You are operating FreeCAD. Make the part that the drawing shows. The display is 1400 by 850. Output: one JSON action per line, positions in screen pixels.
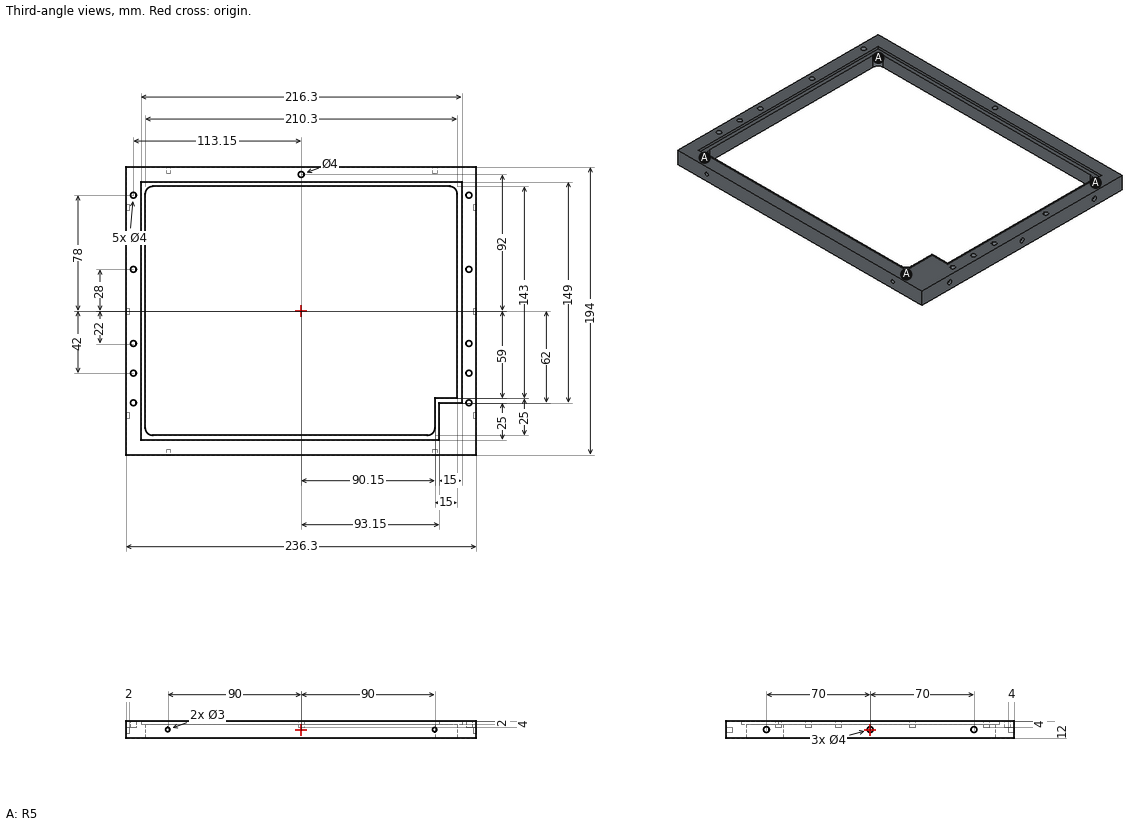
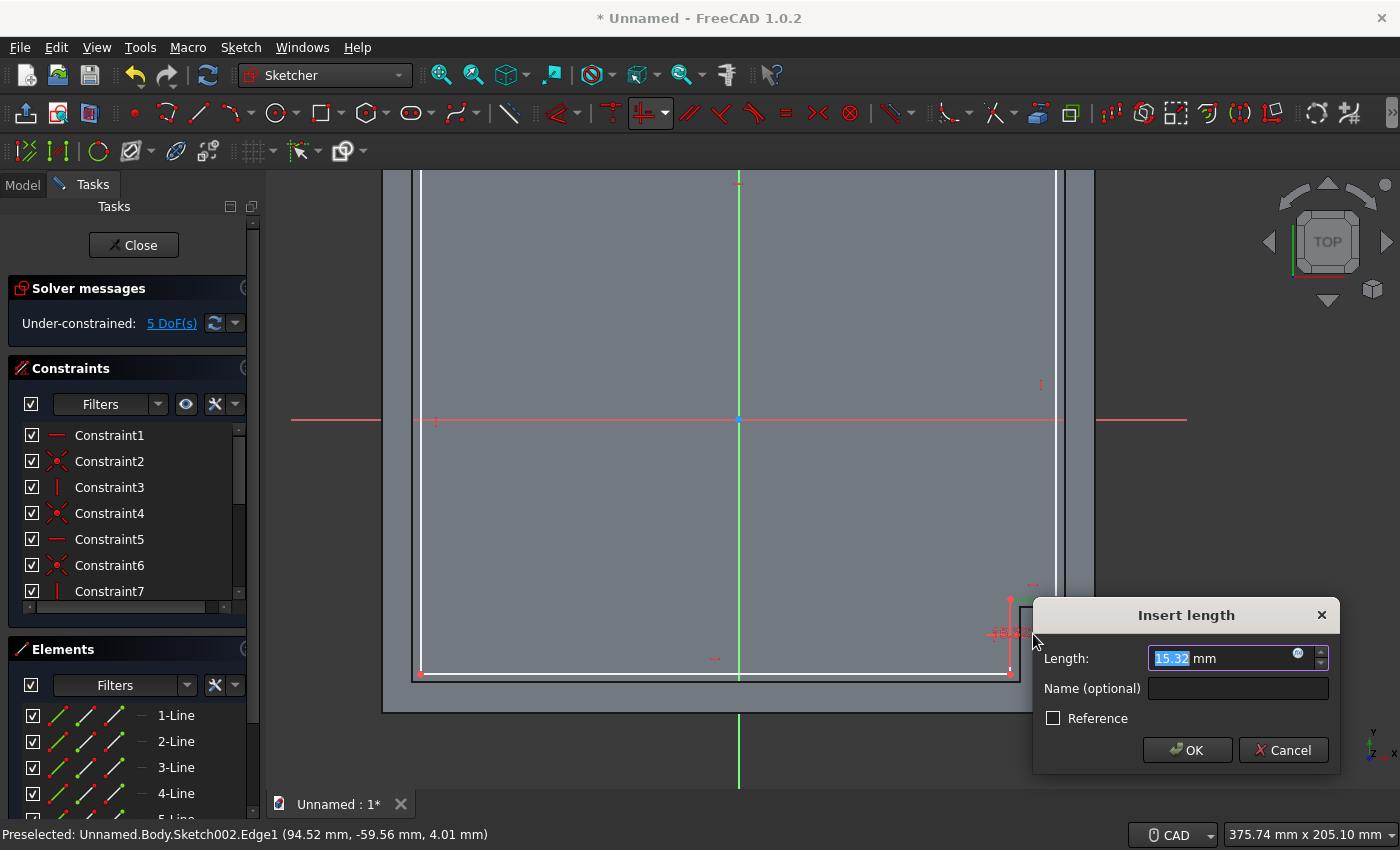
{"action": "type", "text": "15"}
{"action": "key", "text": "Return"}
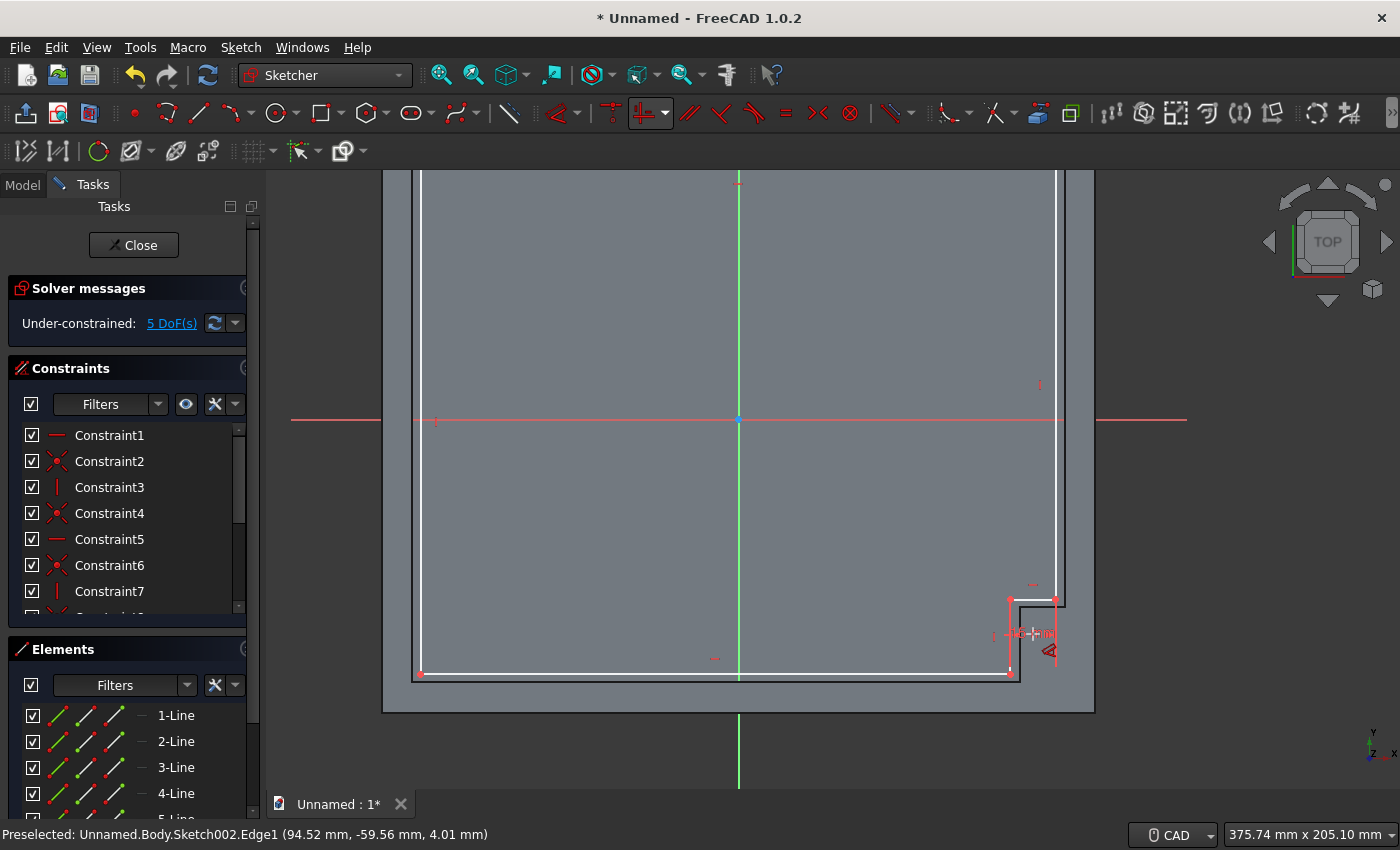
{"action": "left_click", "coordinate": [1010, 652]}
{"action": "left_click", "coordinate": [1044, 654]}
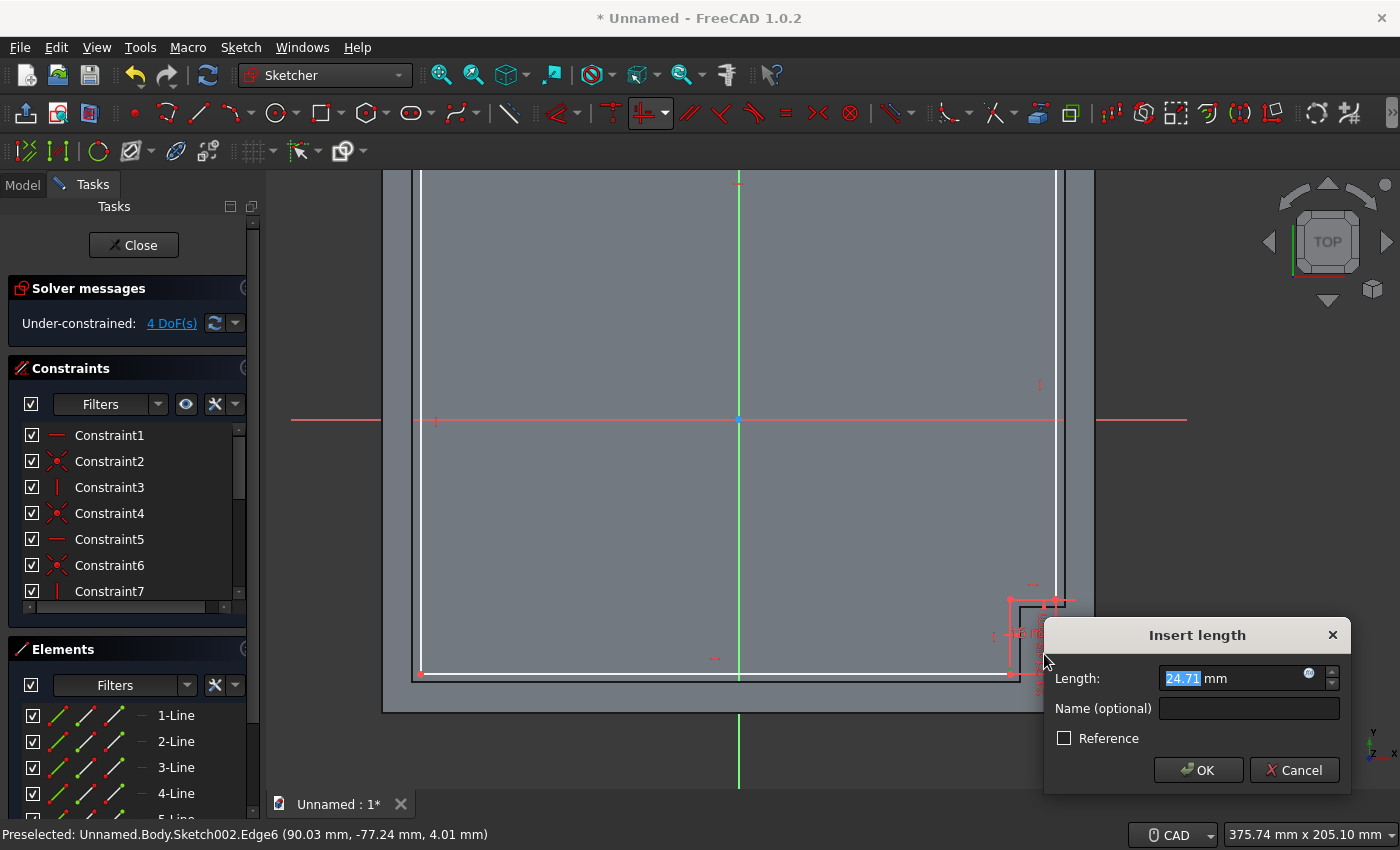
{"action": "type", "text": "25"}
{"action": "key", "text": "Return"}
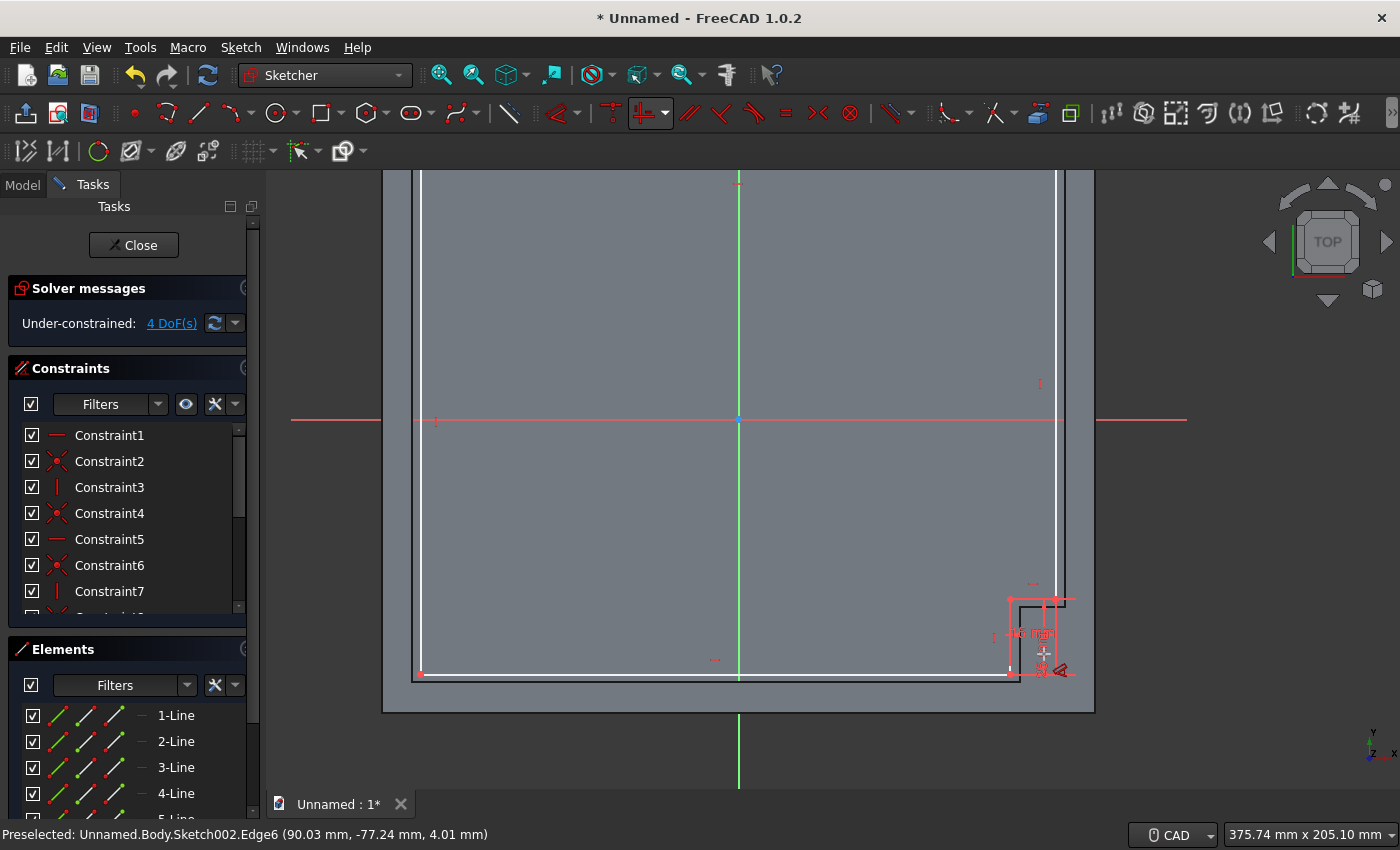
{"action": "left_click", "coordinate": [1056, 470]}
{"action": "left_click", "coordinate": [1090, 399]}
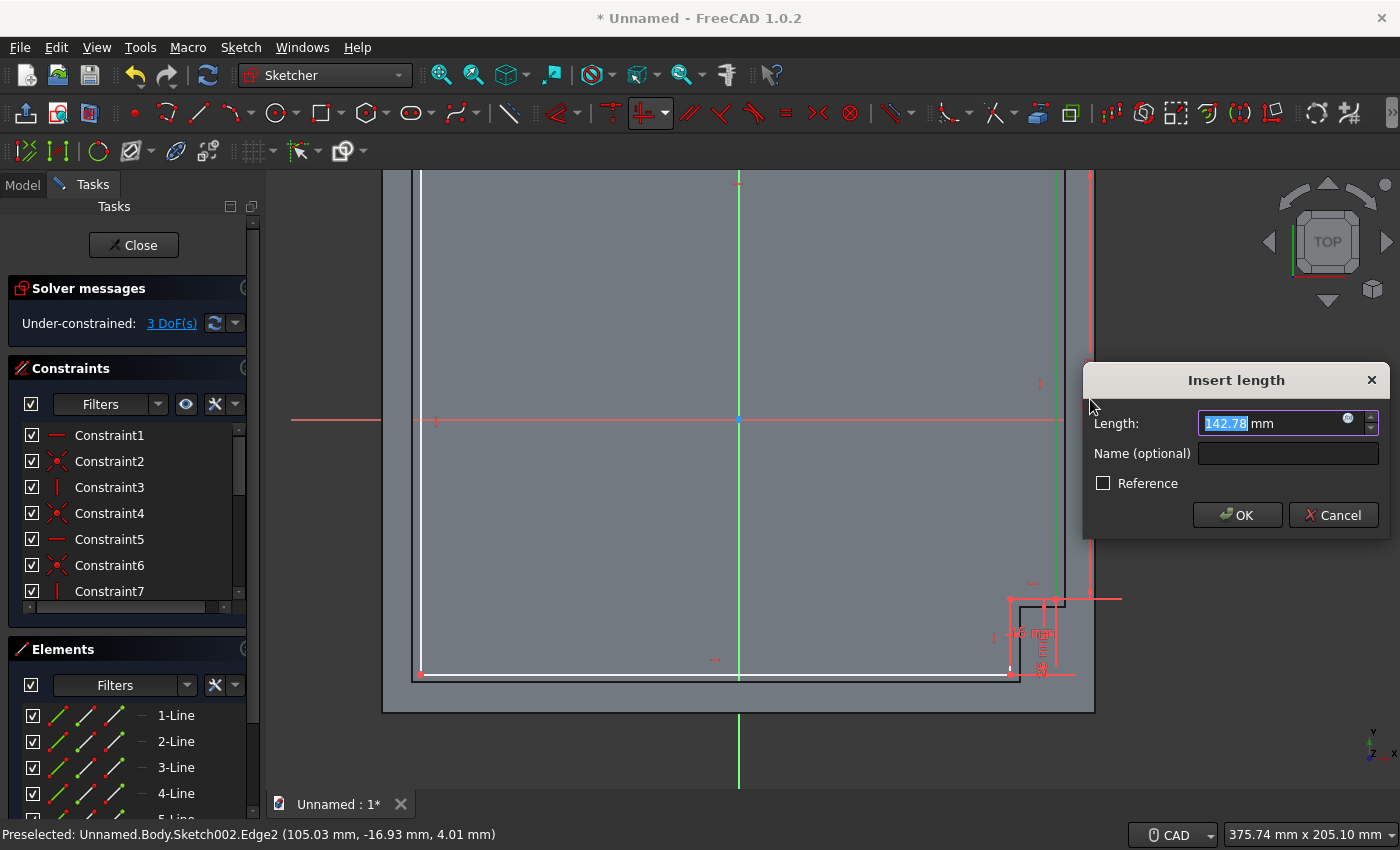
{"action": "type", "text": "143"}
{"action": "key", "text": "Return"}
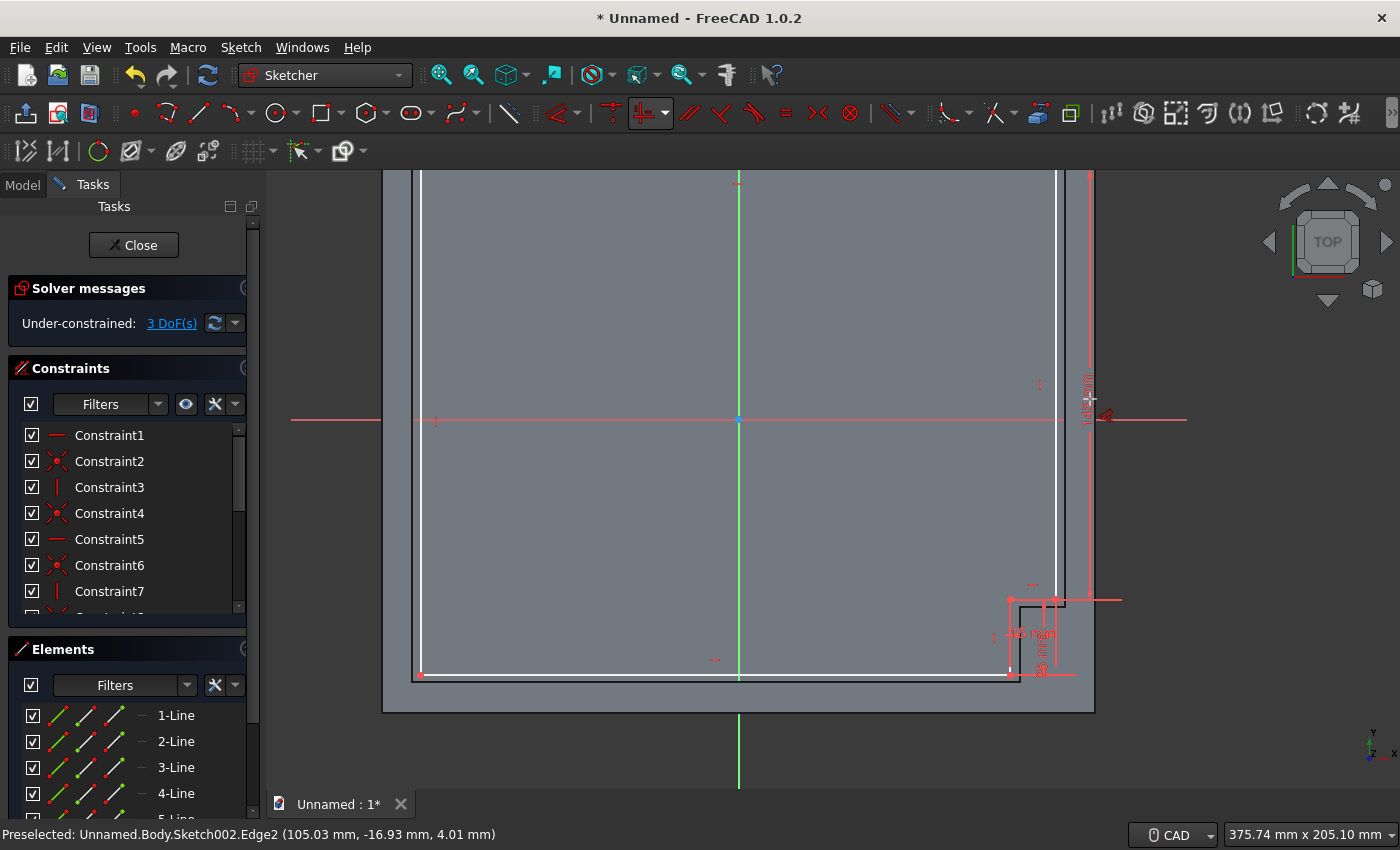
{"action": "left_click", "coordinate": [1010, 600]}
{"action": "left_click", "coordinate": [705, 510]}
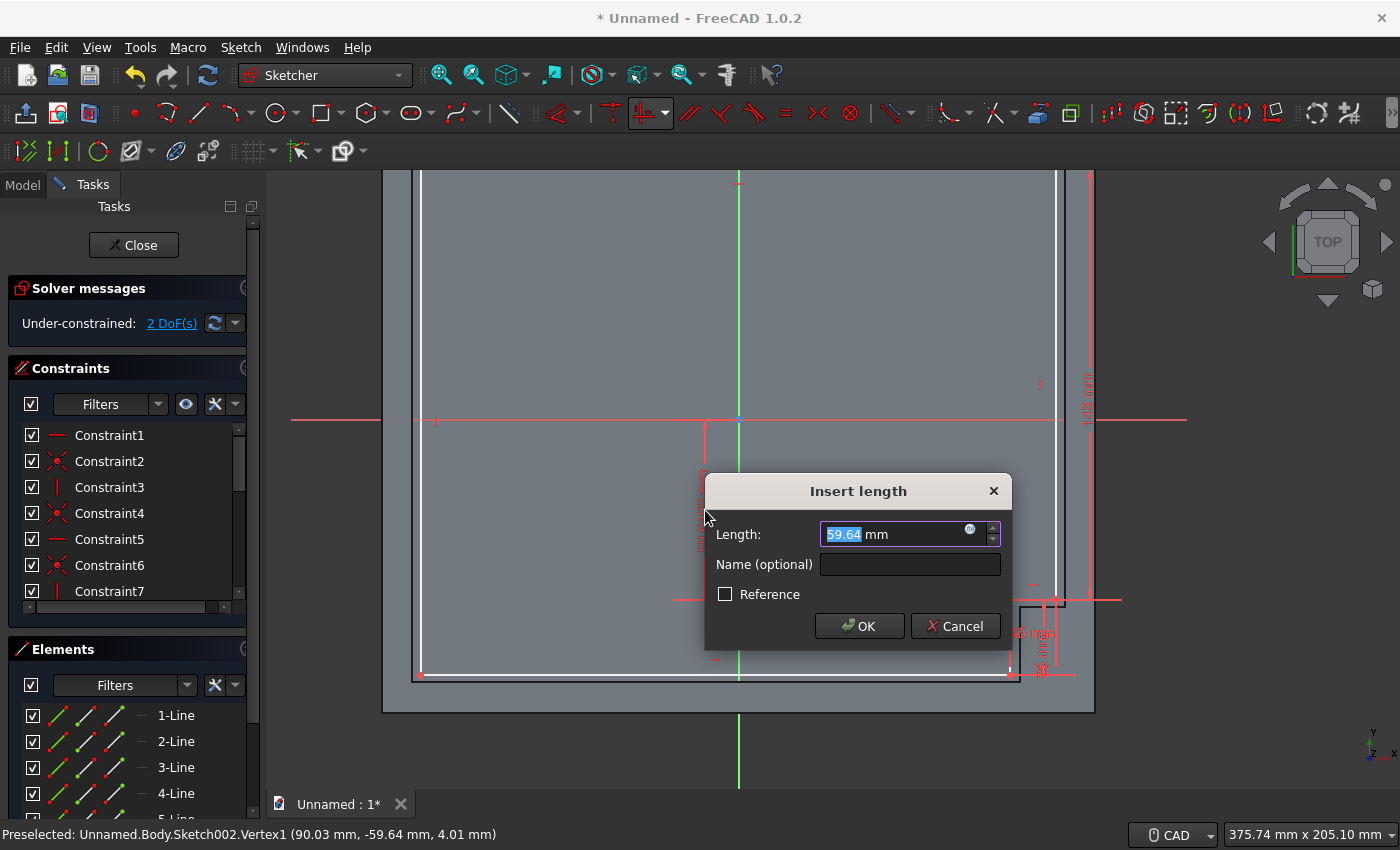
{"action": "type", "text": "59"}
{"action": "key", "text": "Return"}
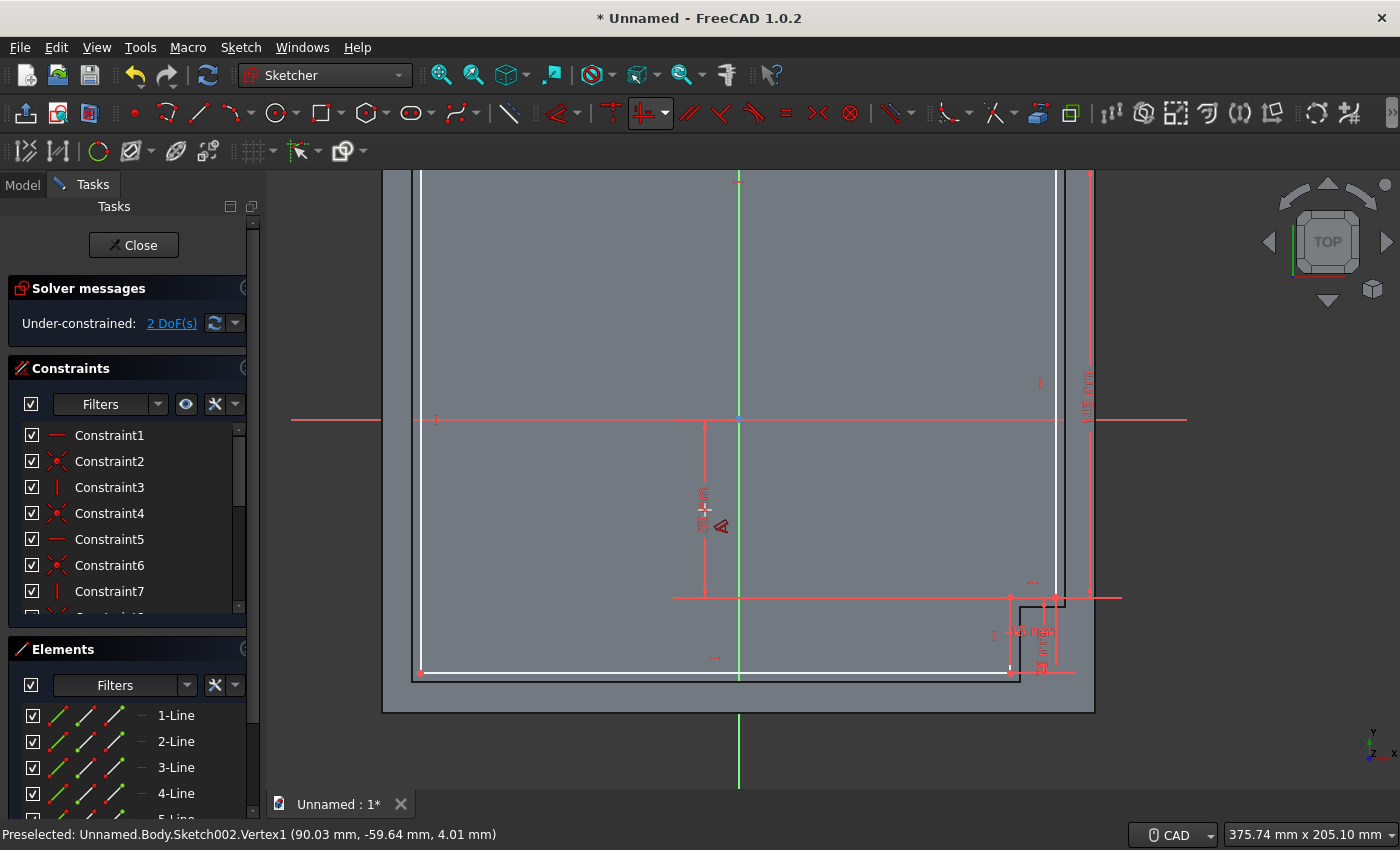
{"action": "scroll", "coordinate": [881, 749], "scroll_direction": "down", "scroll_amount": 1}